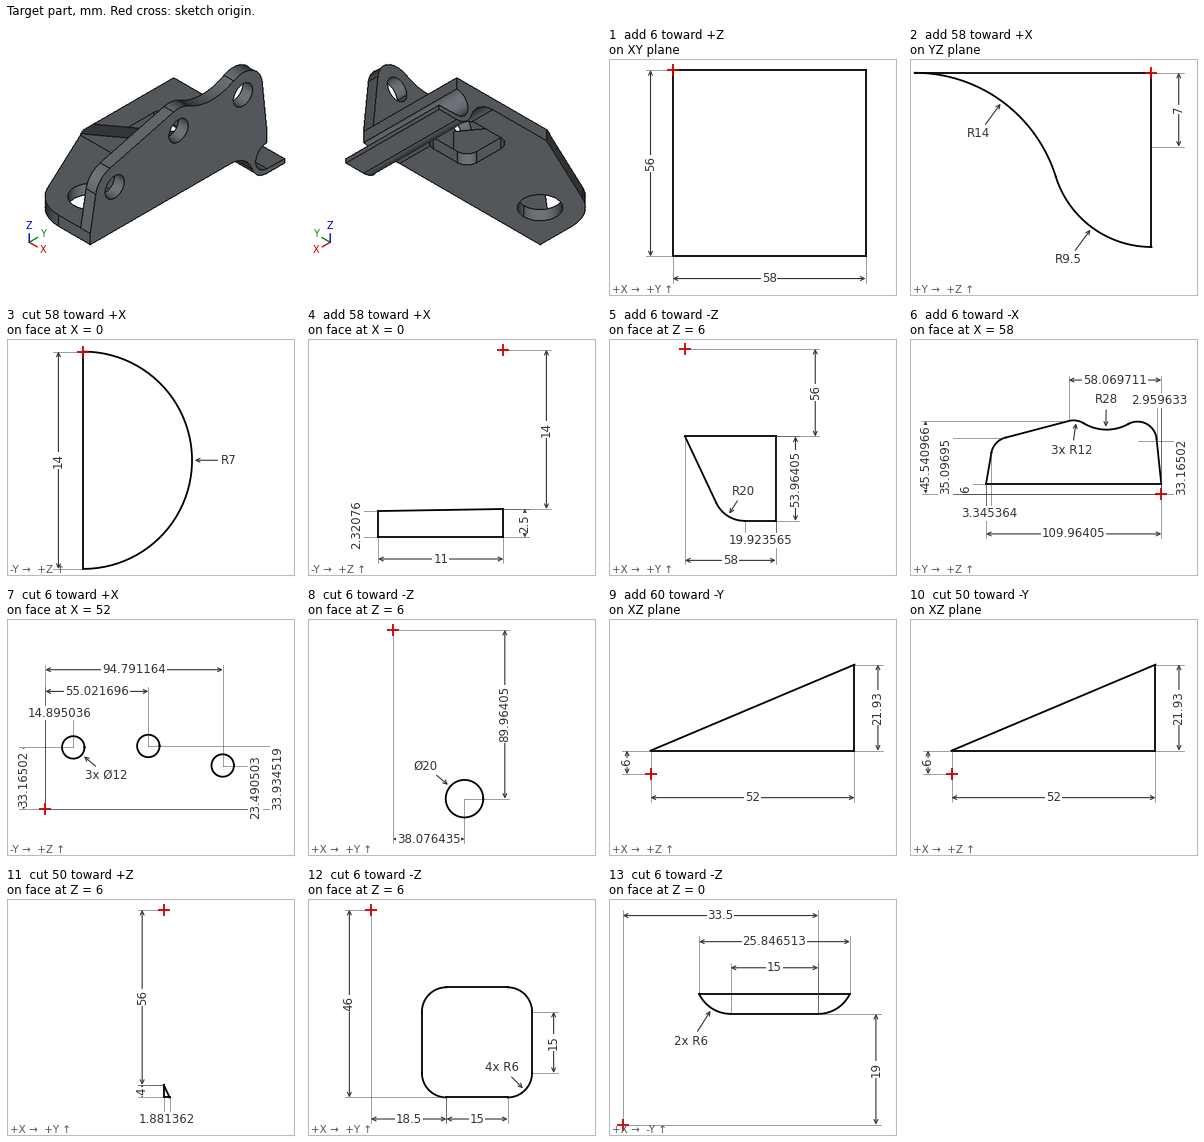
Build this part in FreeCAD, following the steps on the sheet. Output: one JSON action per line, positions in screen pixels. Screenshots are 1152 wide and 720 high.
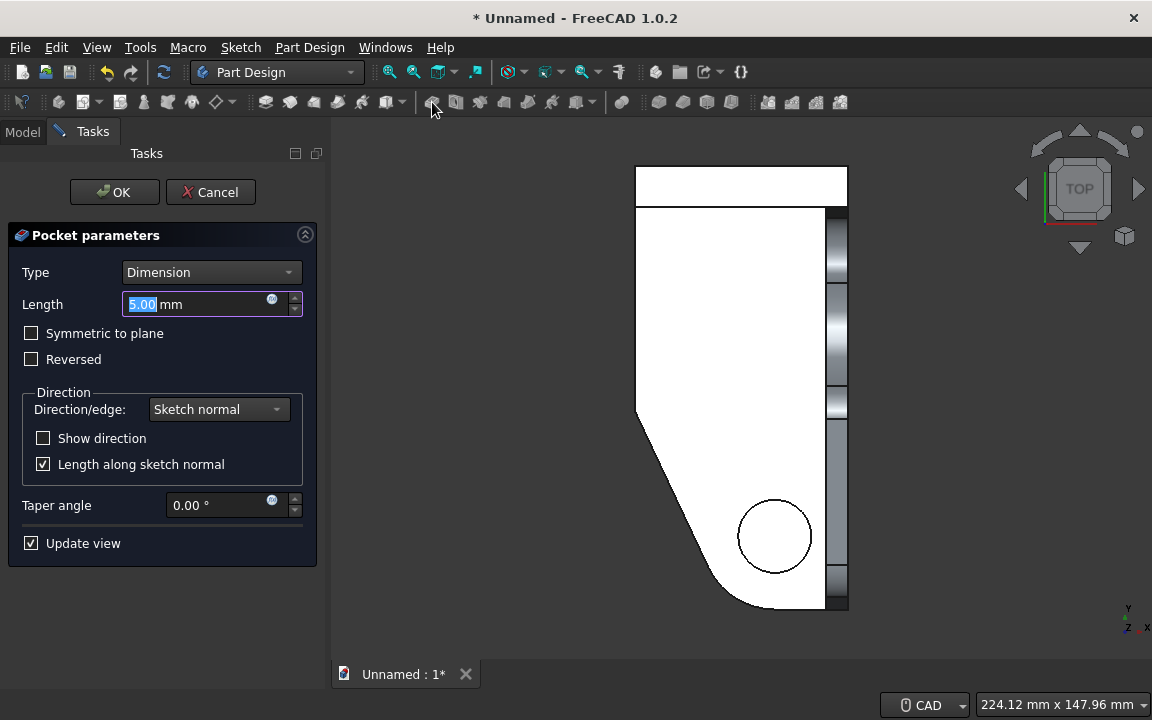
{"action": "type", "text": "6"}
{"action": "key", "text": "Tab"}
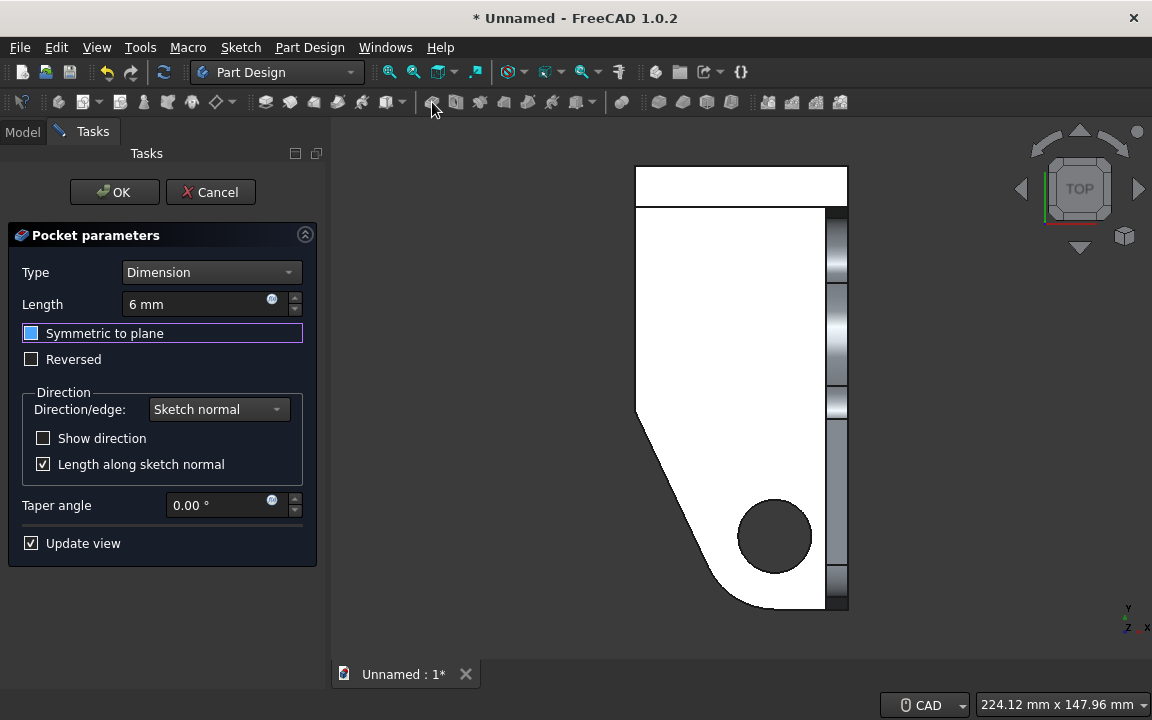
{"action": "left_click", "coordinate": [115, 192]}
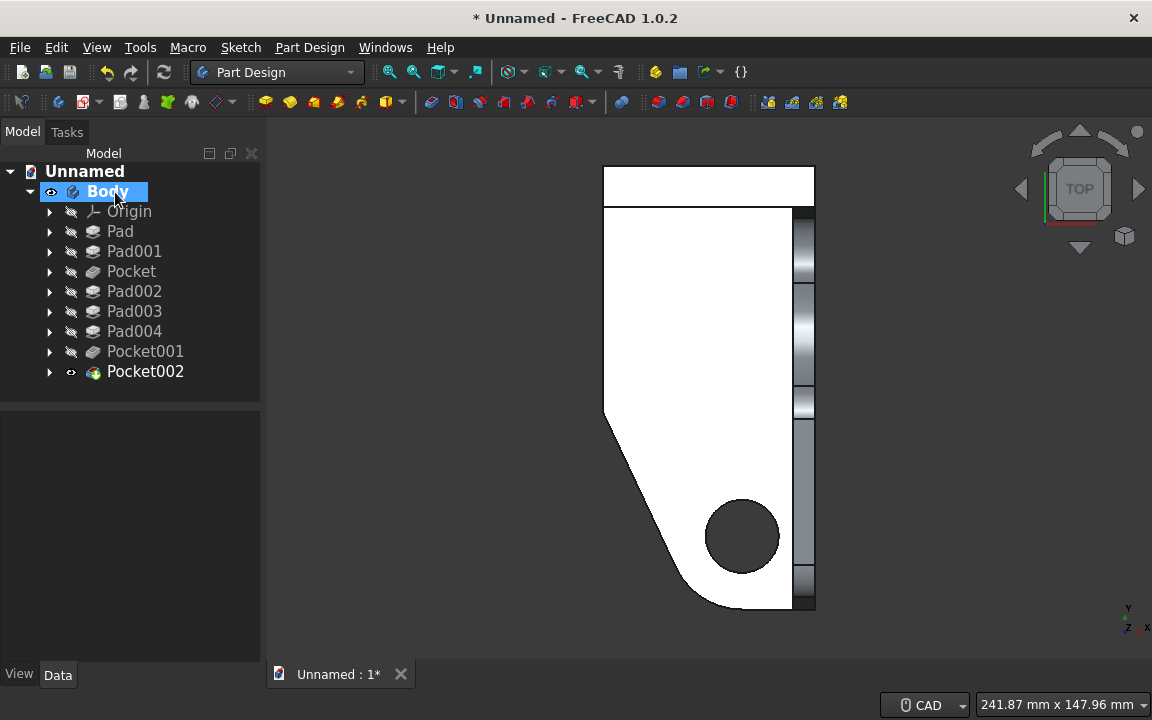
{"action": "left_click", "coordinate": [84, 102]}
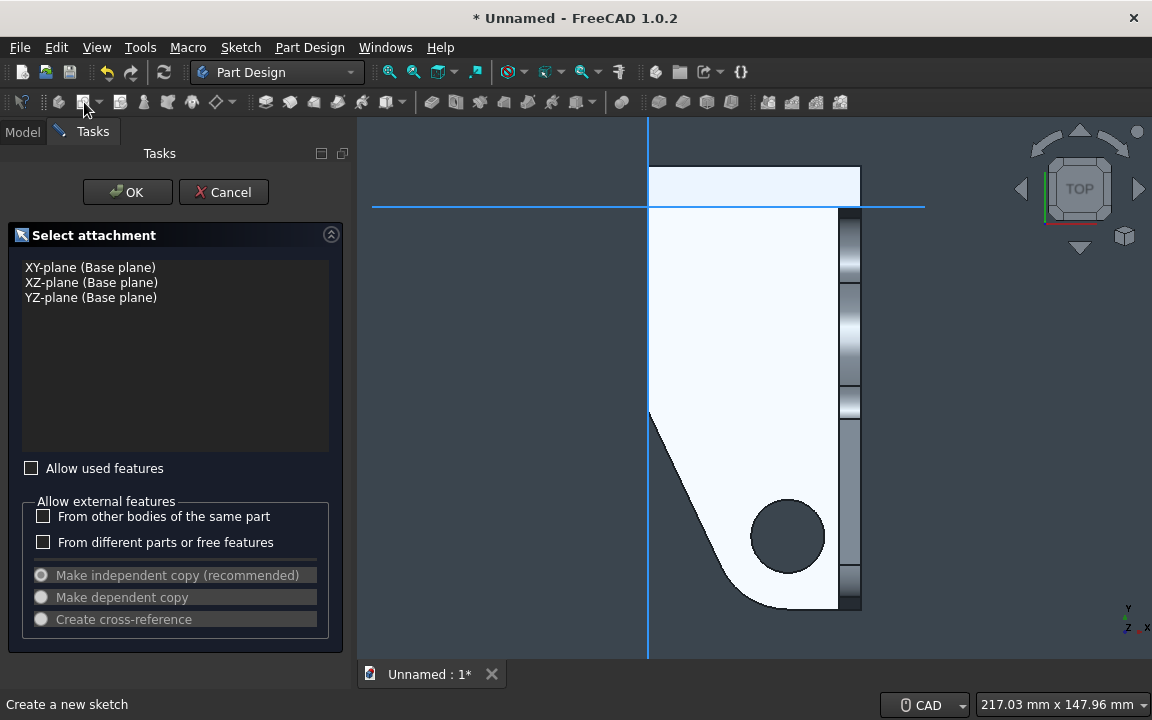
{"action": "left_click", "coordinate": [82, 282]}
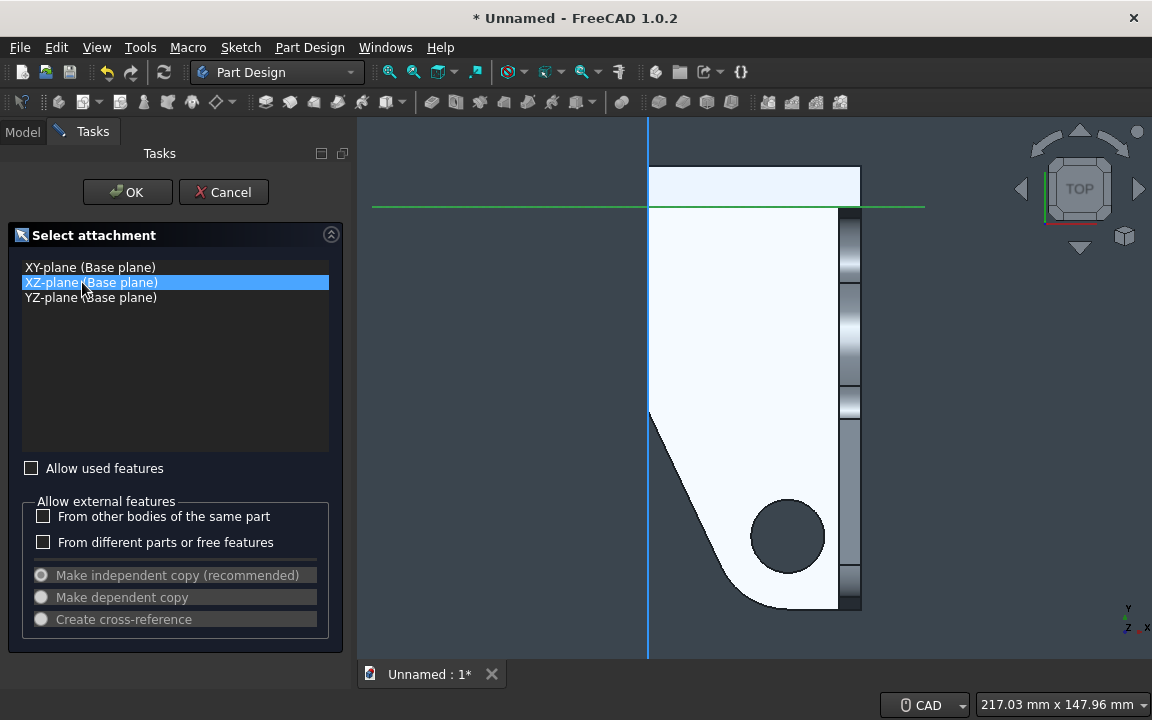
{"action": "left_click", "coordinate": [128, 192]}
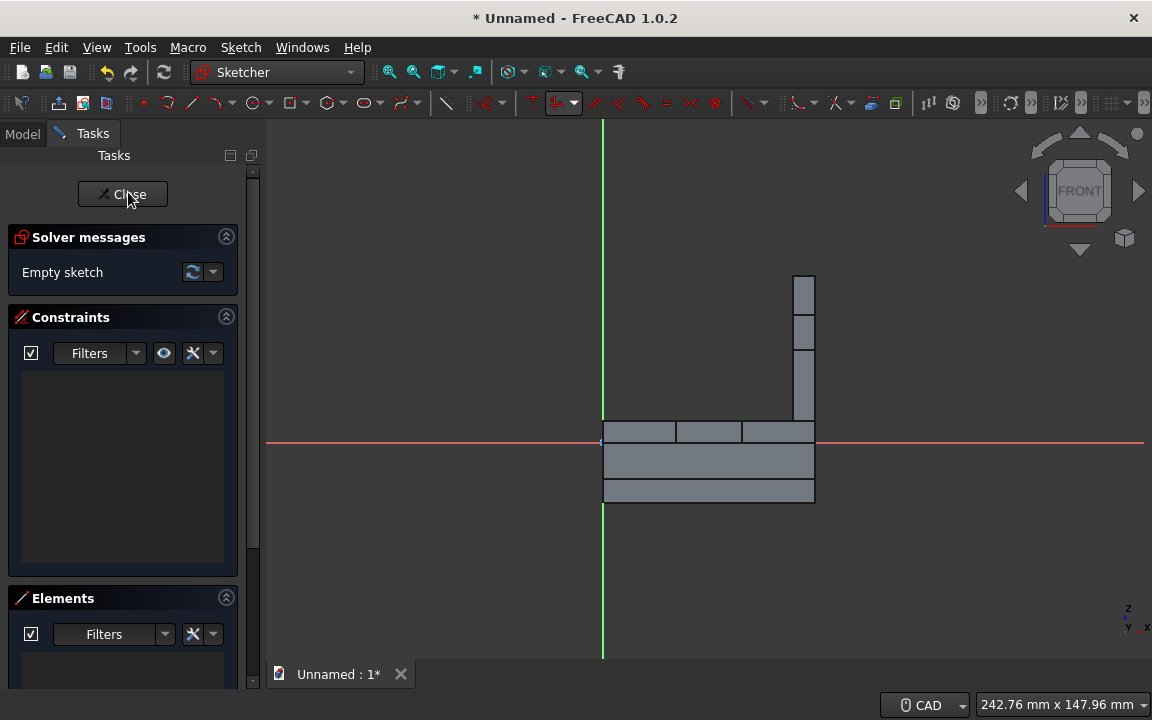
{"action": "left_click", "coordinate": [108, 104]}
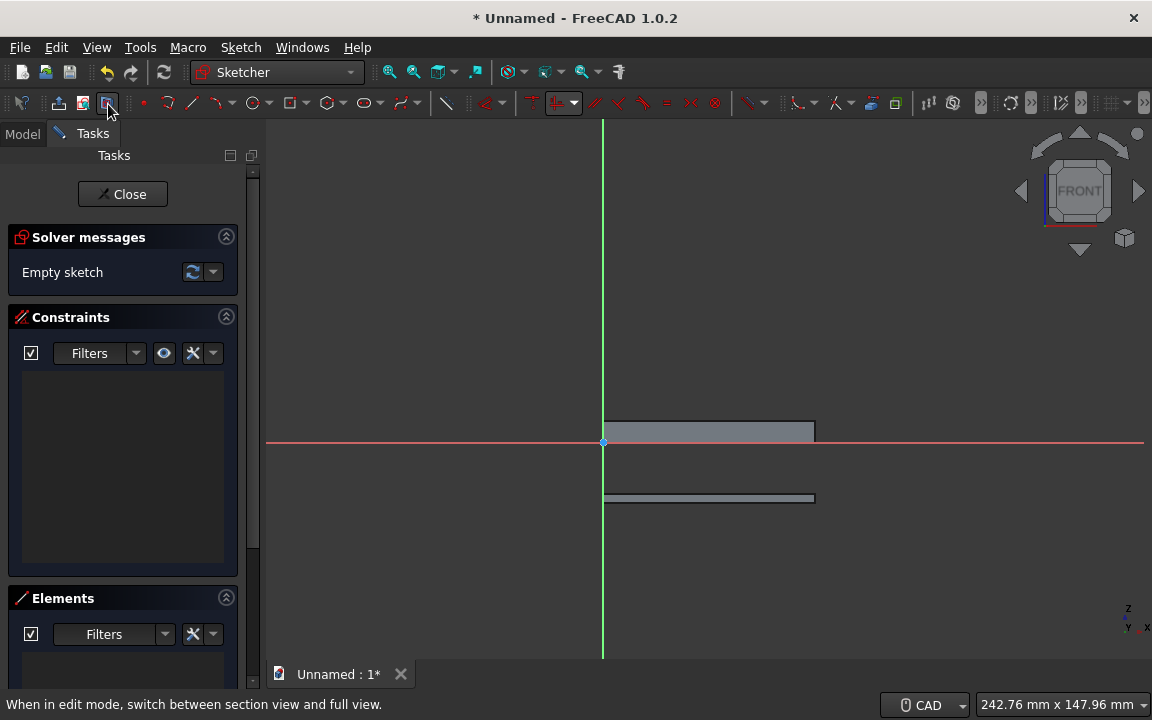
{"action": "scroll", "coordinate": [732, 393], "scroll_direction": "up", "scroll_amount": 5}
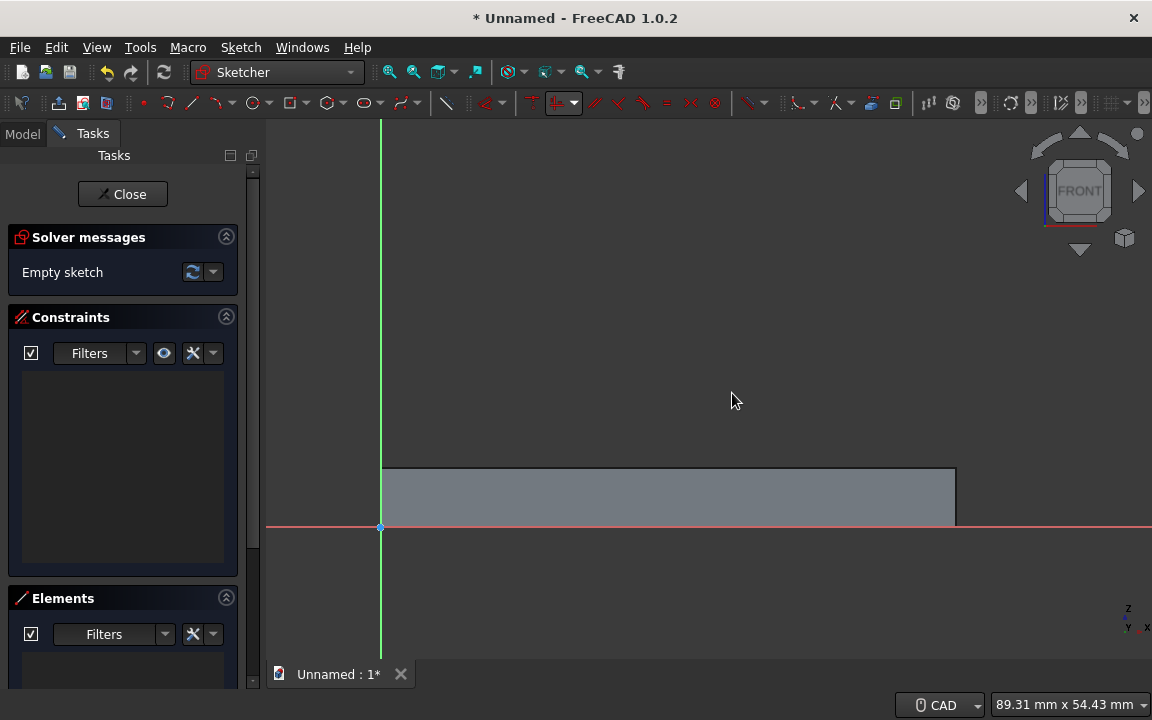
{"action": "key", "text": "g m"}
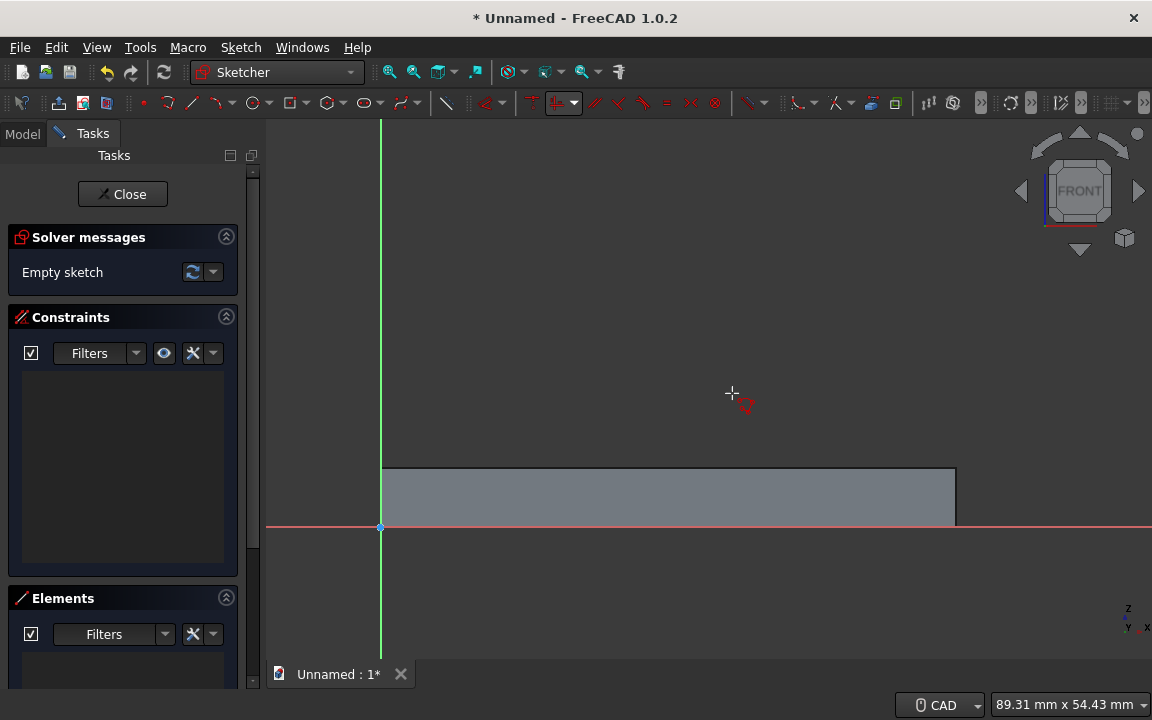
{"action": "left_click", "coordinate": [381, 468]}
{"action": "left_click", "coordinate": [897, 250]}
{"action": "left_click", "coordinate": [897, 468]}
{"action": "left_click", "coordinate": [381, 469]}
{"action": "key", "text": "Escape"}
{"action": "key", "text": "Escape"}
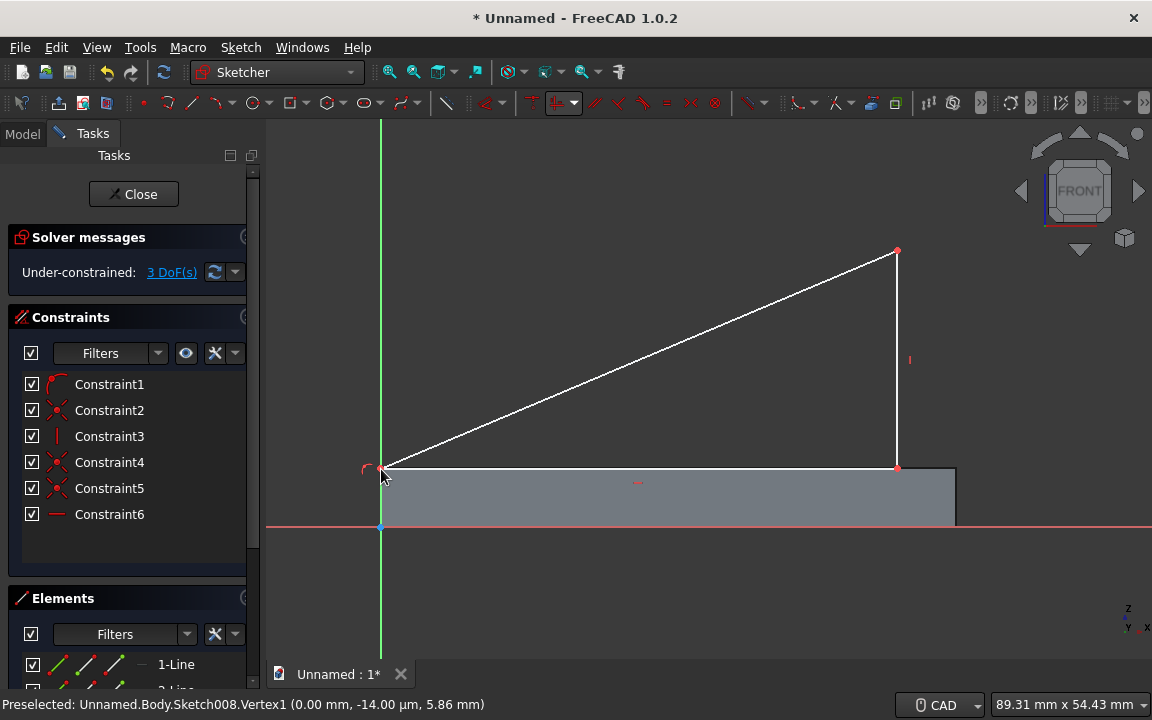
{"action": "left_click", "coordinate": [486, 104]}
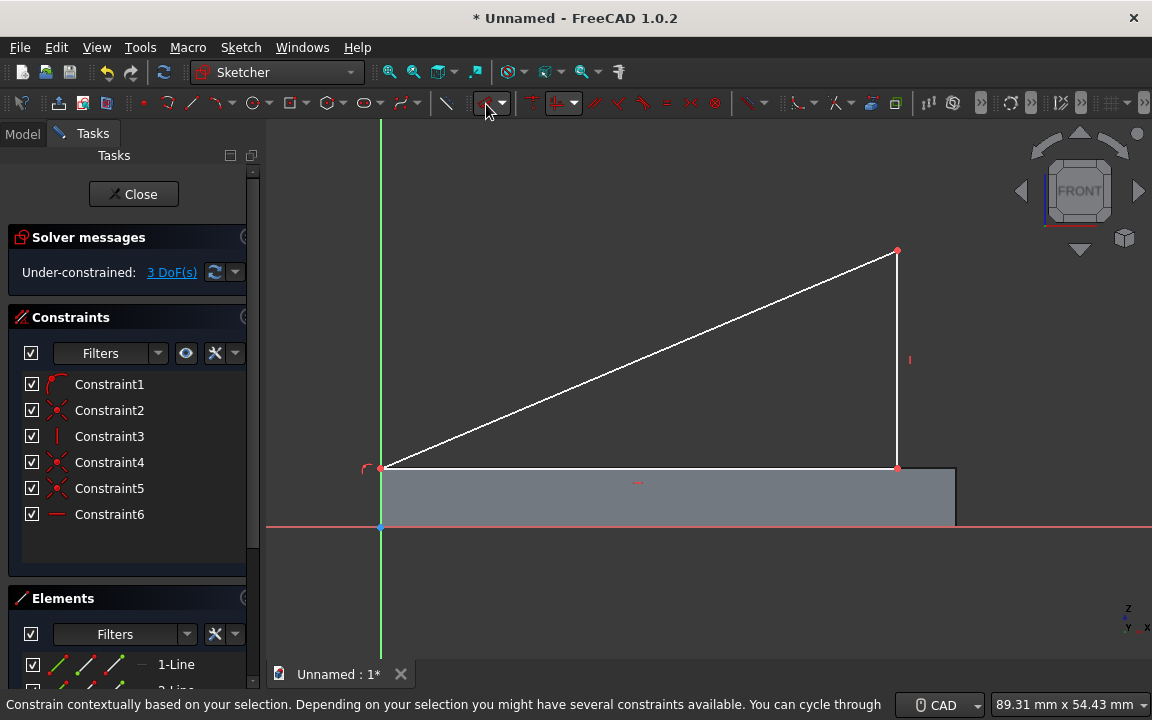
{"action": "left_click", "coordinate": [742, 469]}
{"action": "left_click", "coordinate": [639, 503]}